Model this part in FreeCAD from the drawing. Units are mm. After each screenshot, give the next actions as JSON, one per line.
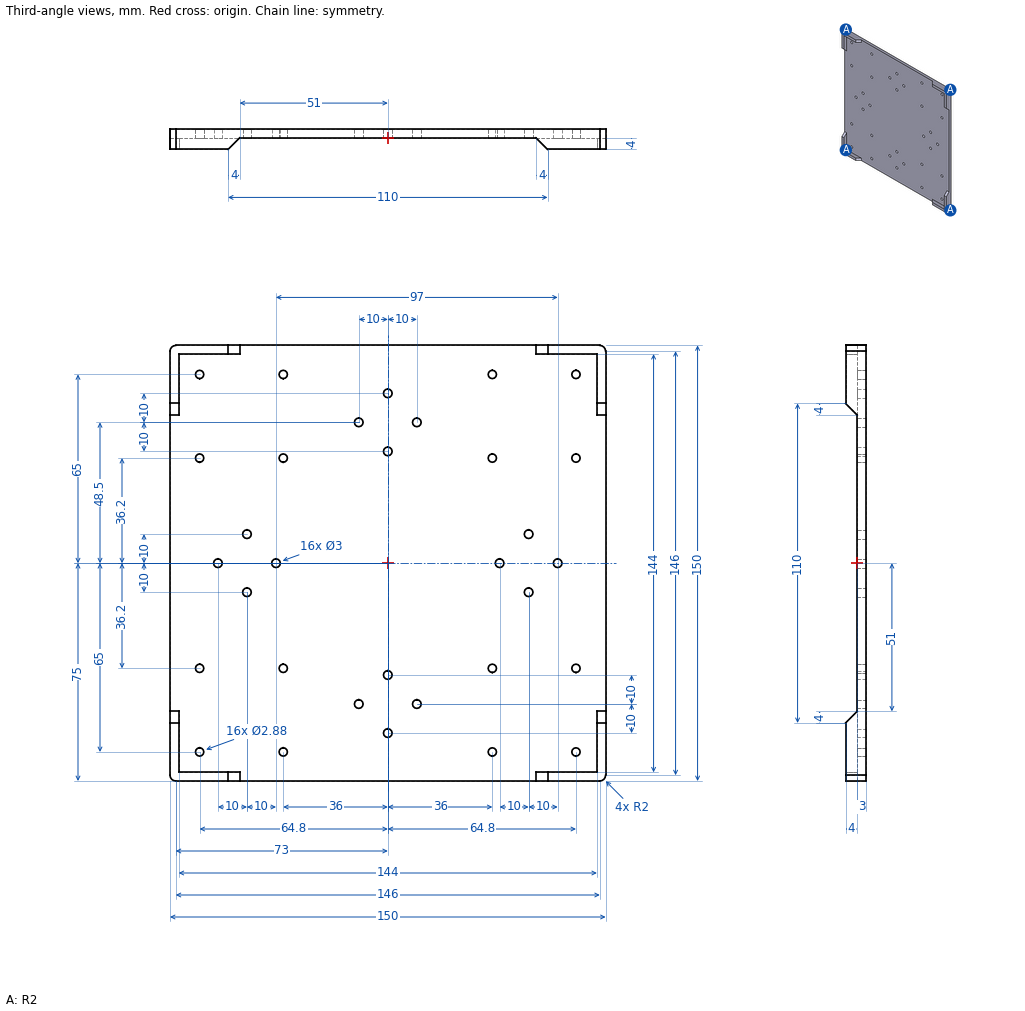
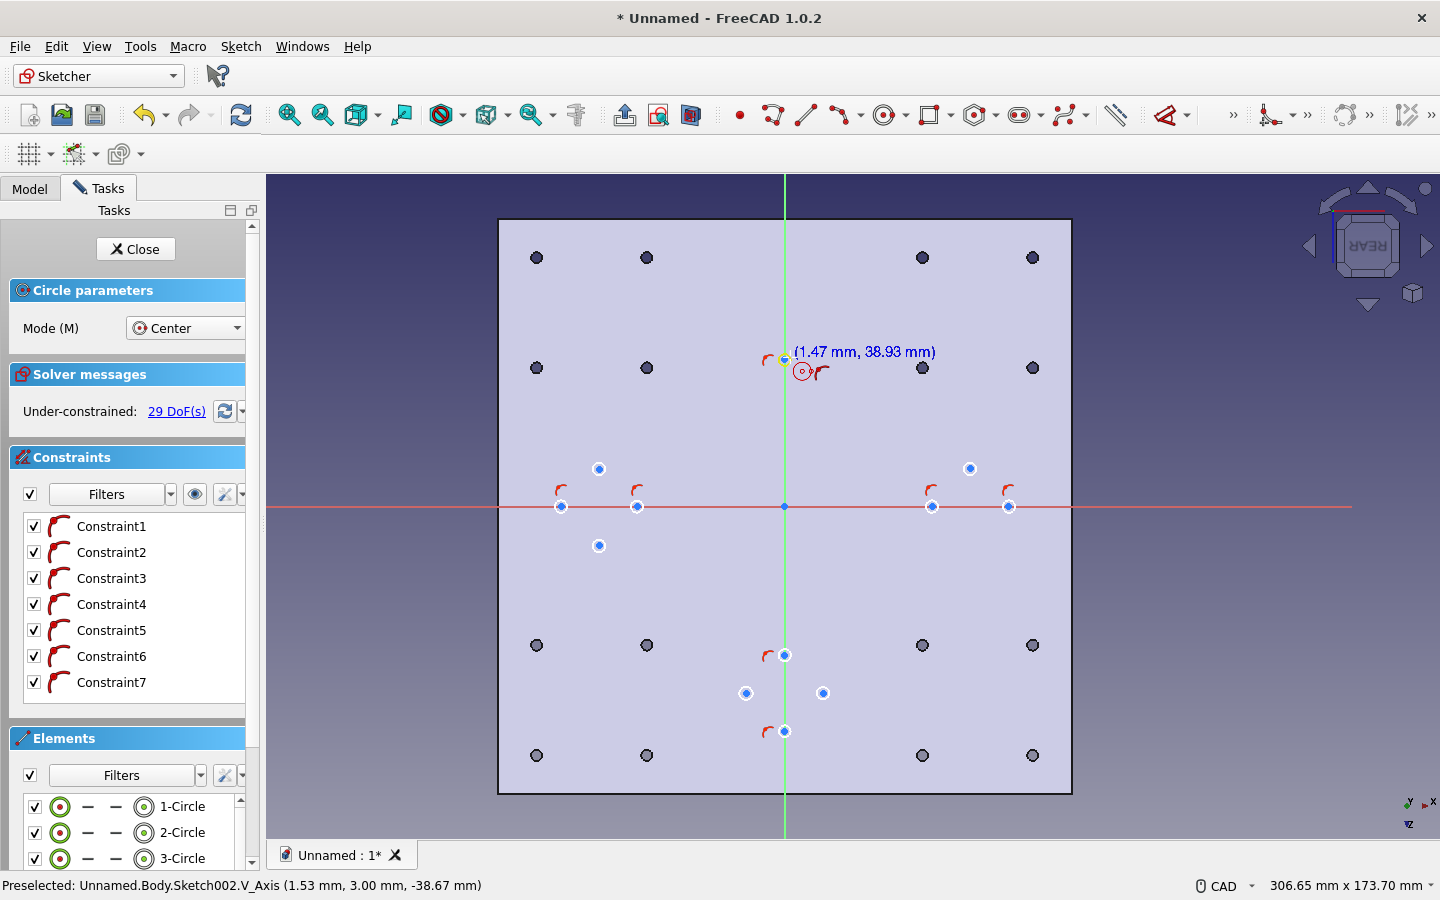
{"action": "left_click", "coordinate": [823, 321]}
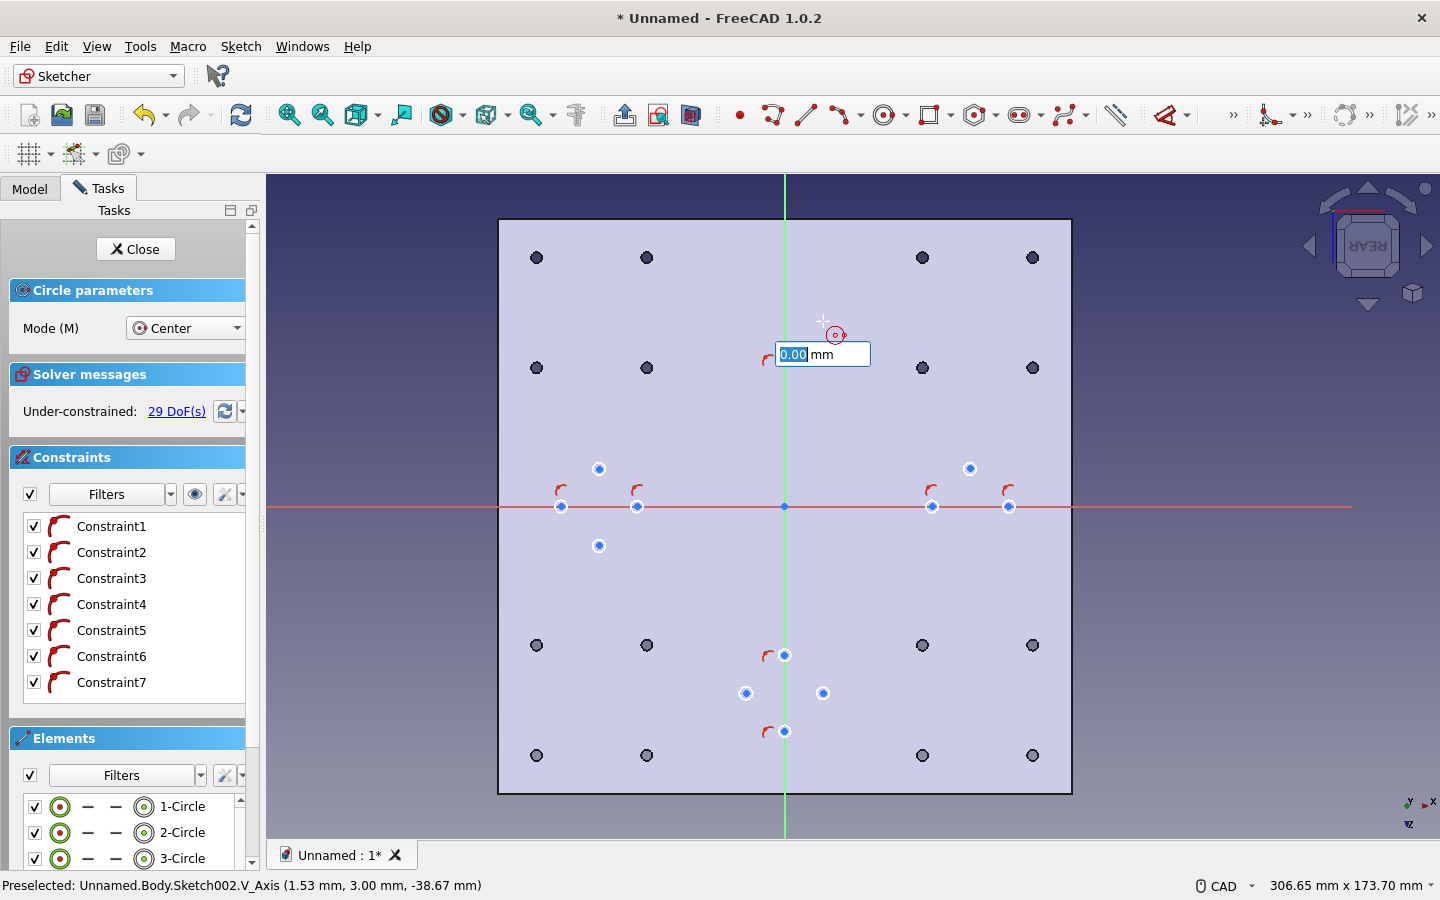
{"action": "scroll", "coordinate": [827, 317], "scroll_direction": "up", "scroll_amount": 6}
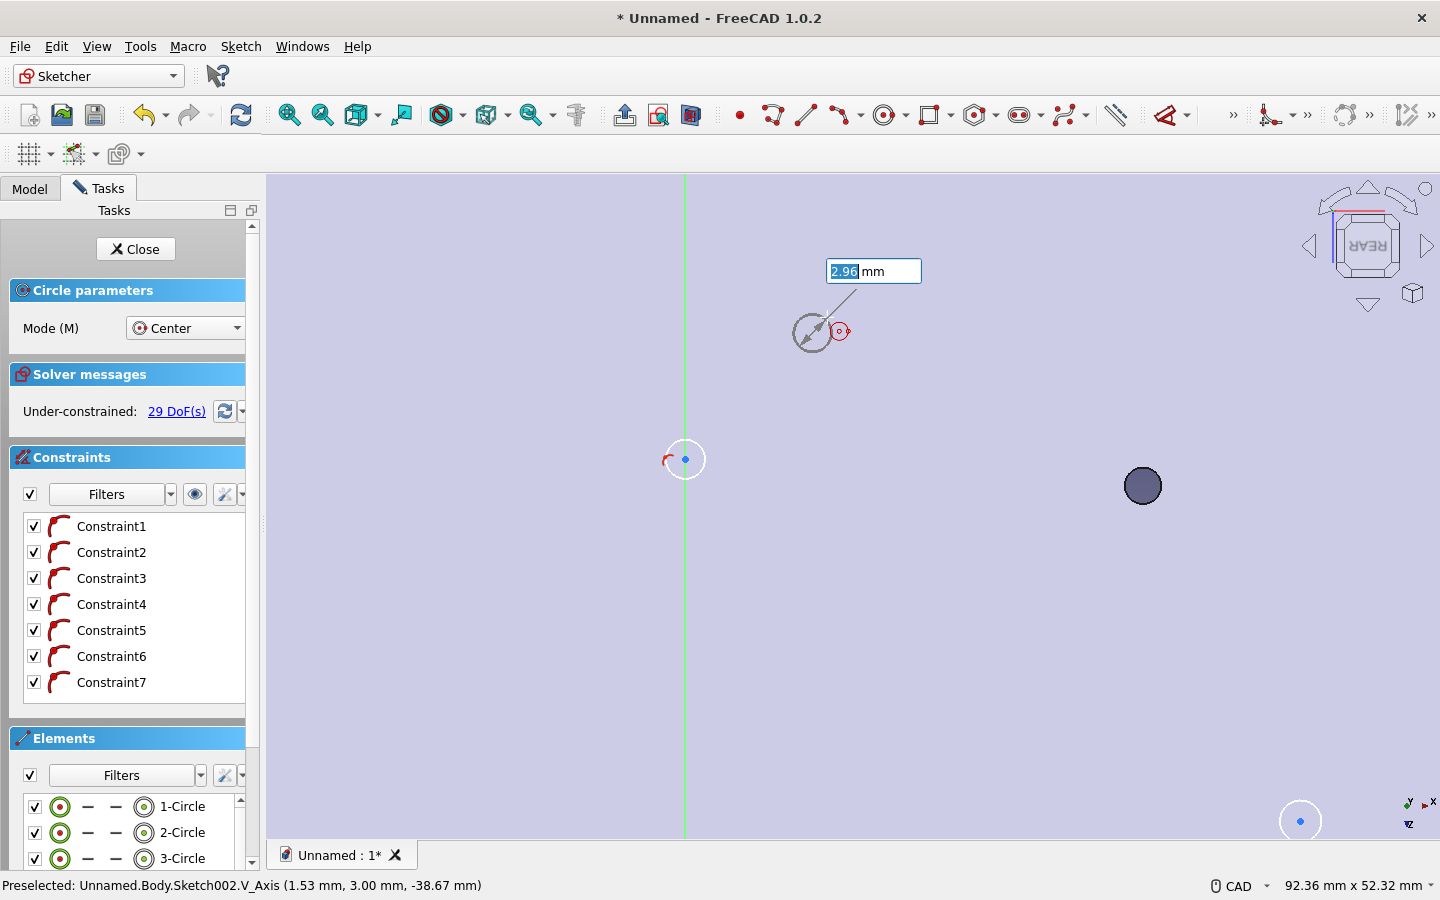
{"action": "left_click", "coordinate": [826, 316]}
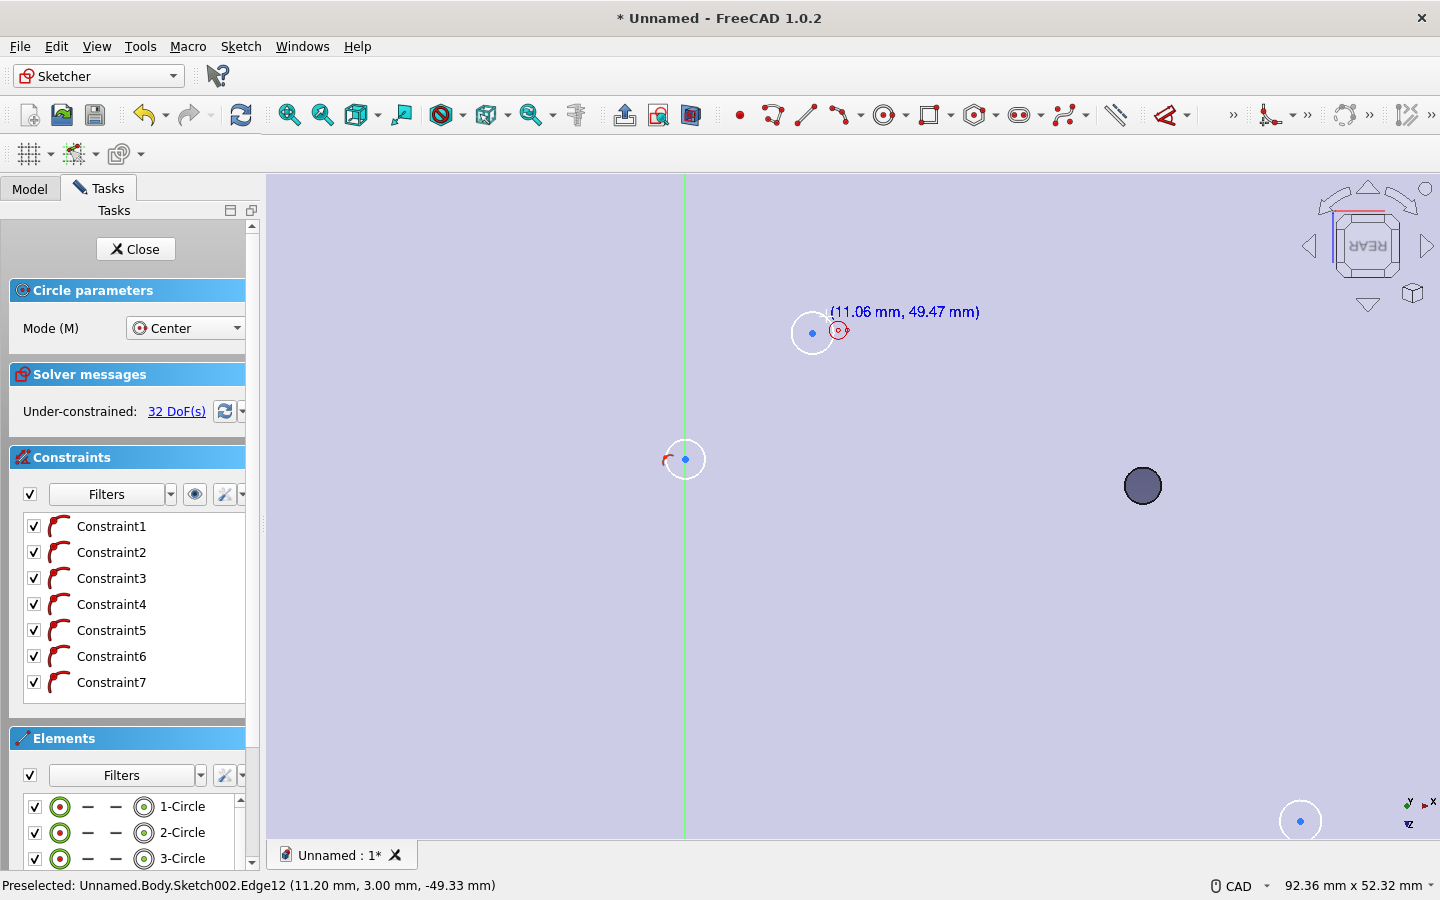
{"action": "scroll", "coordinate": [827, 317], "scroll_direction": "down", "scroll_amount": 6}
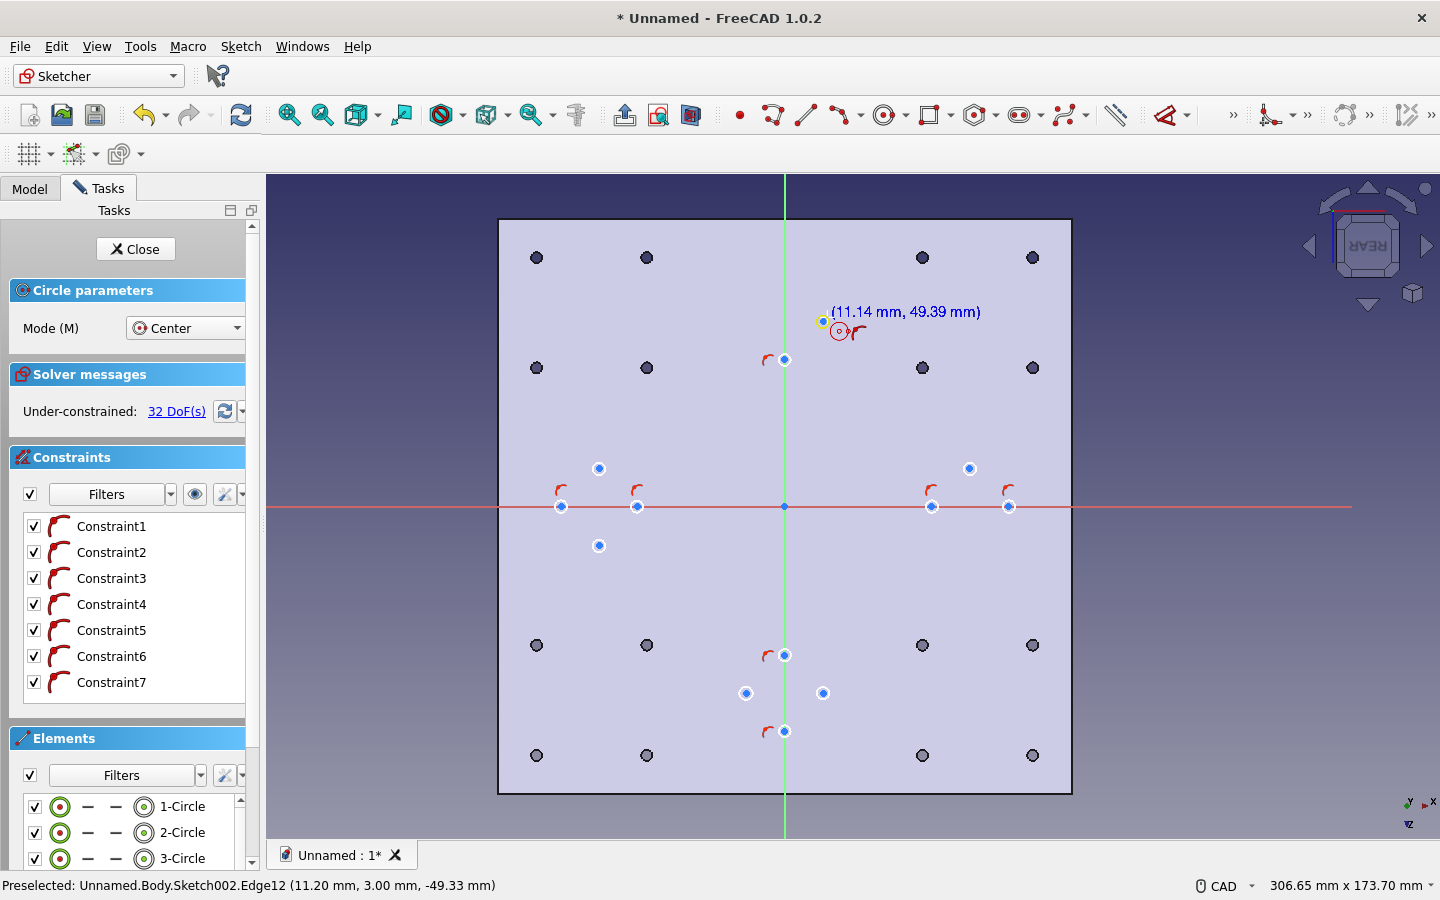
{"action": "left_click", "coordinate": [785, 283]}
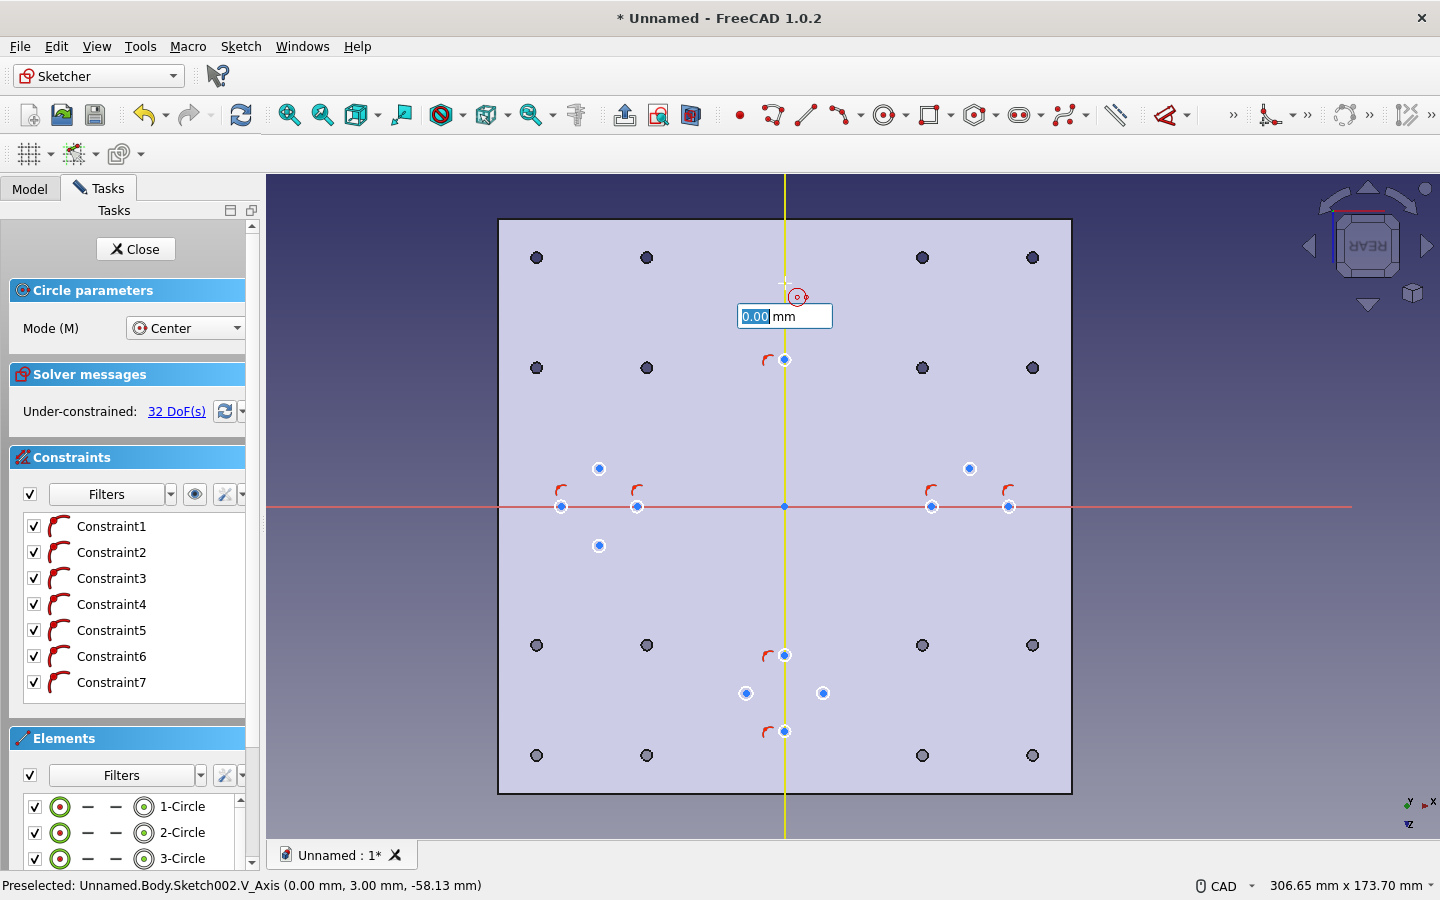
{"action": "scroll", "coordinate": [790, 281], "scroll_direction": "up", "scroll_amount": 6}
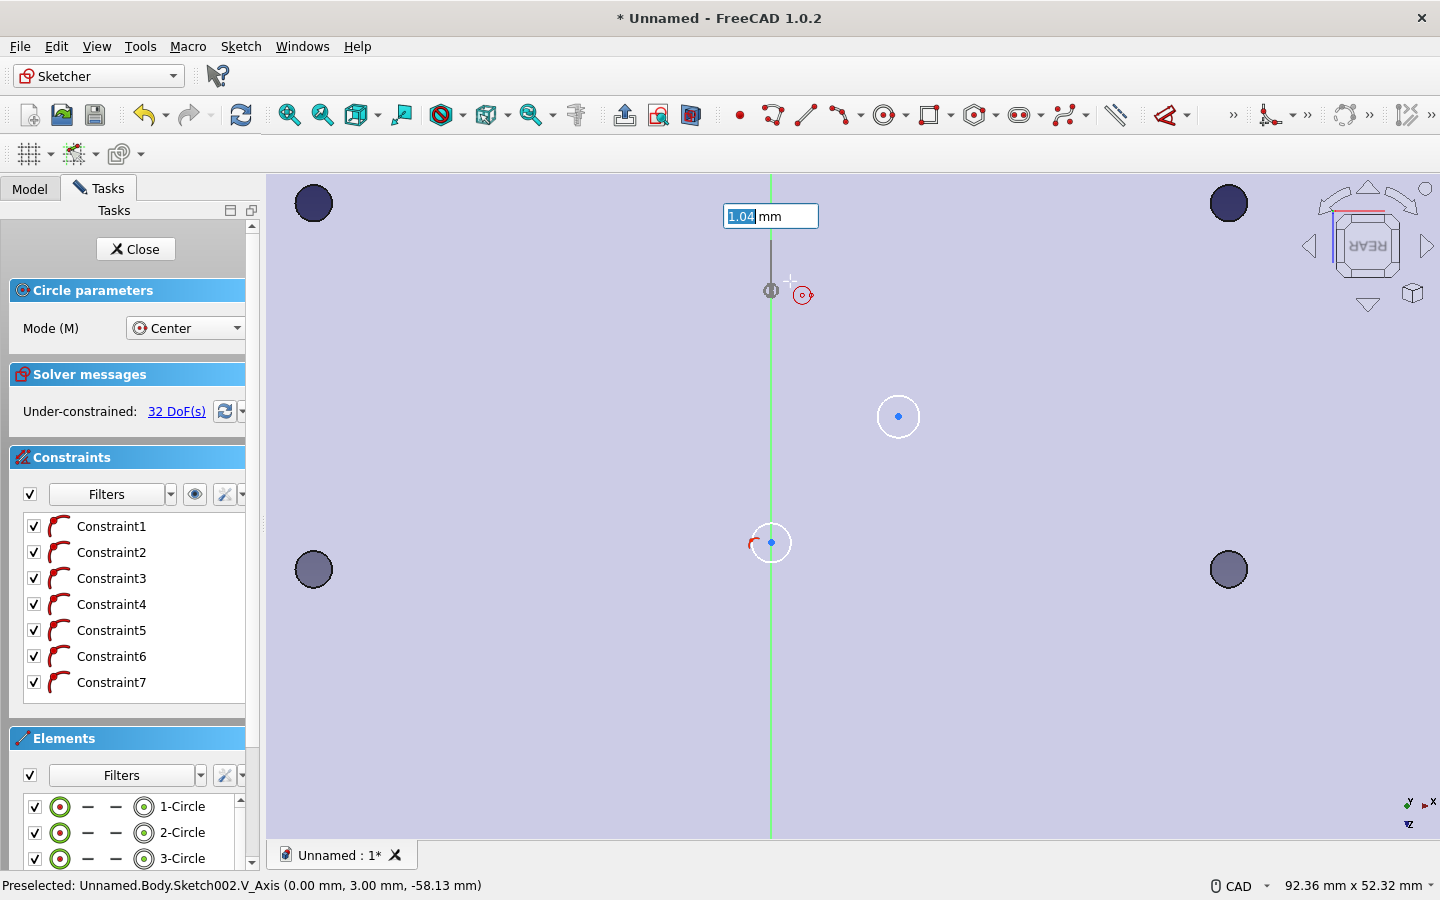
{"action": "left_click", "coordinate": [789, 279]}